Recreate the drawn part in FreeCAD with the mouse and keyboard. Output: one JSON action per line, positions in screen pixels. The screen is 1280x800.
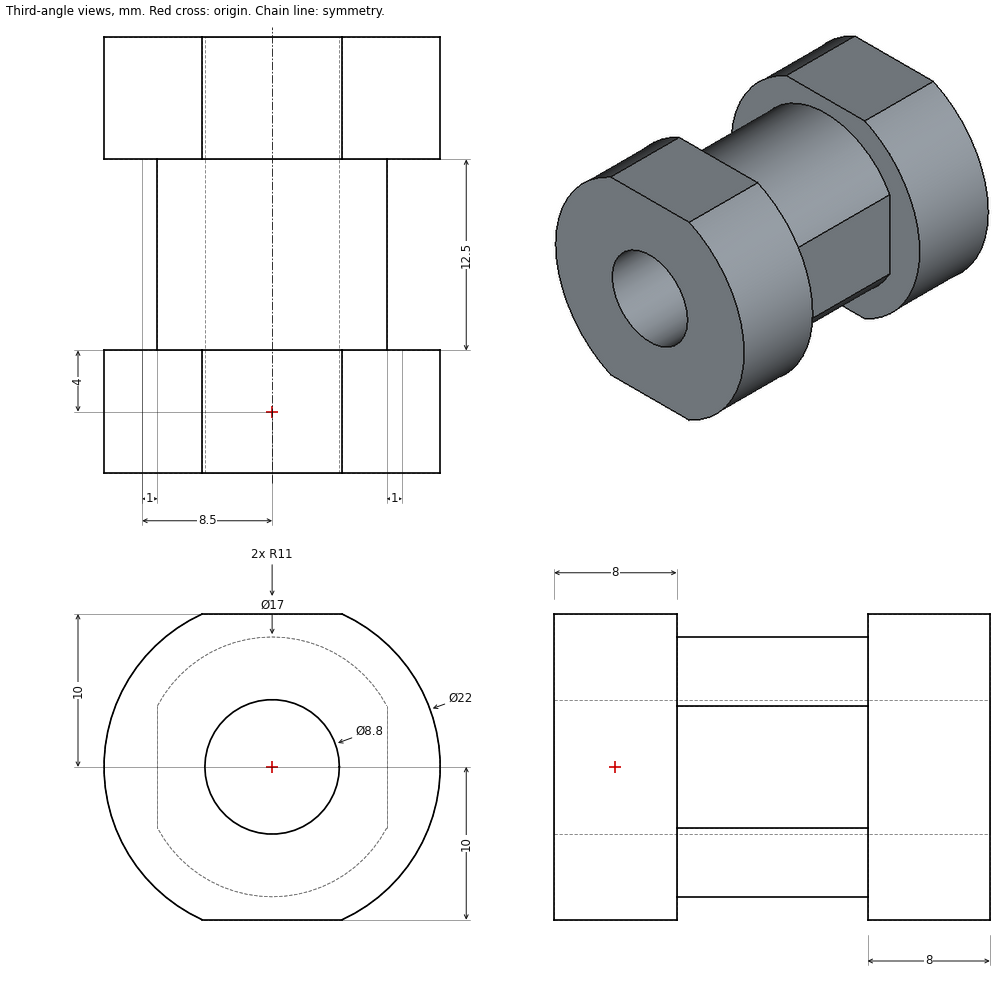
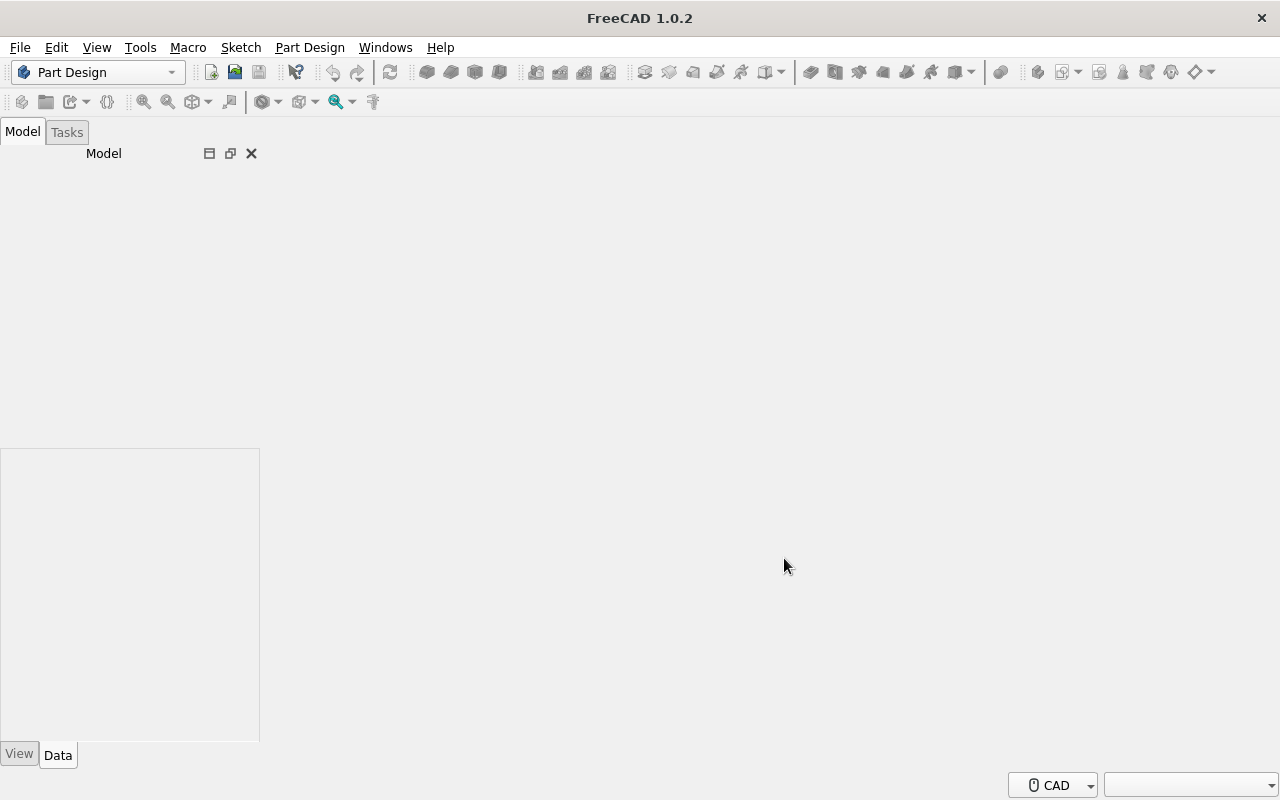
{"action": "left_click", "coordinate": [212, 72]}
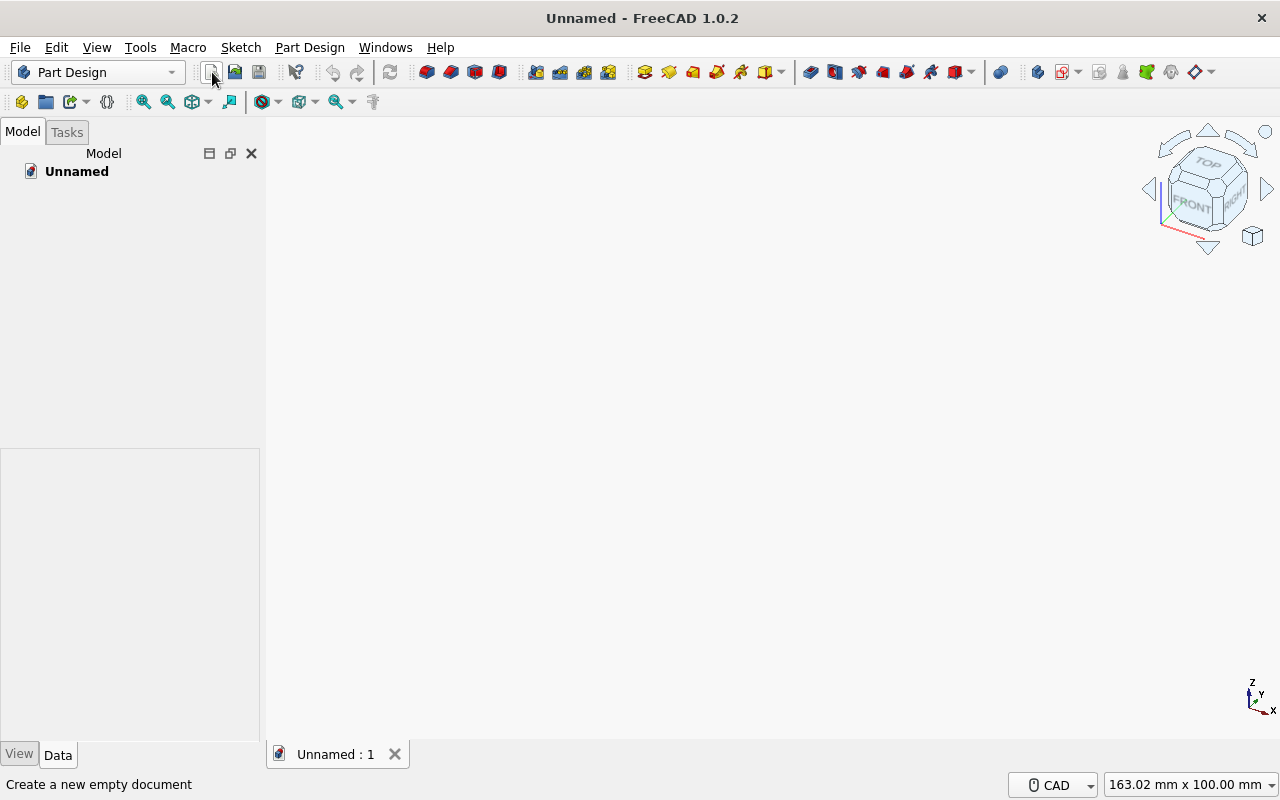
{"action": "left_click", "coordinate": [1062, 72]}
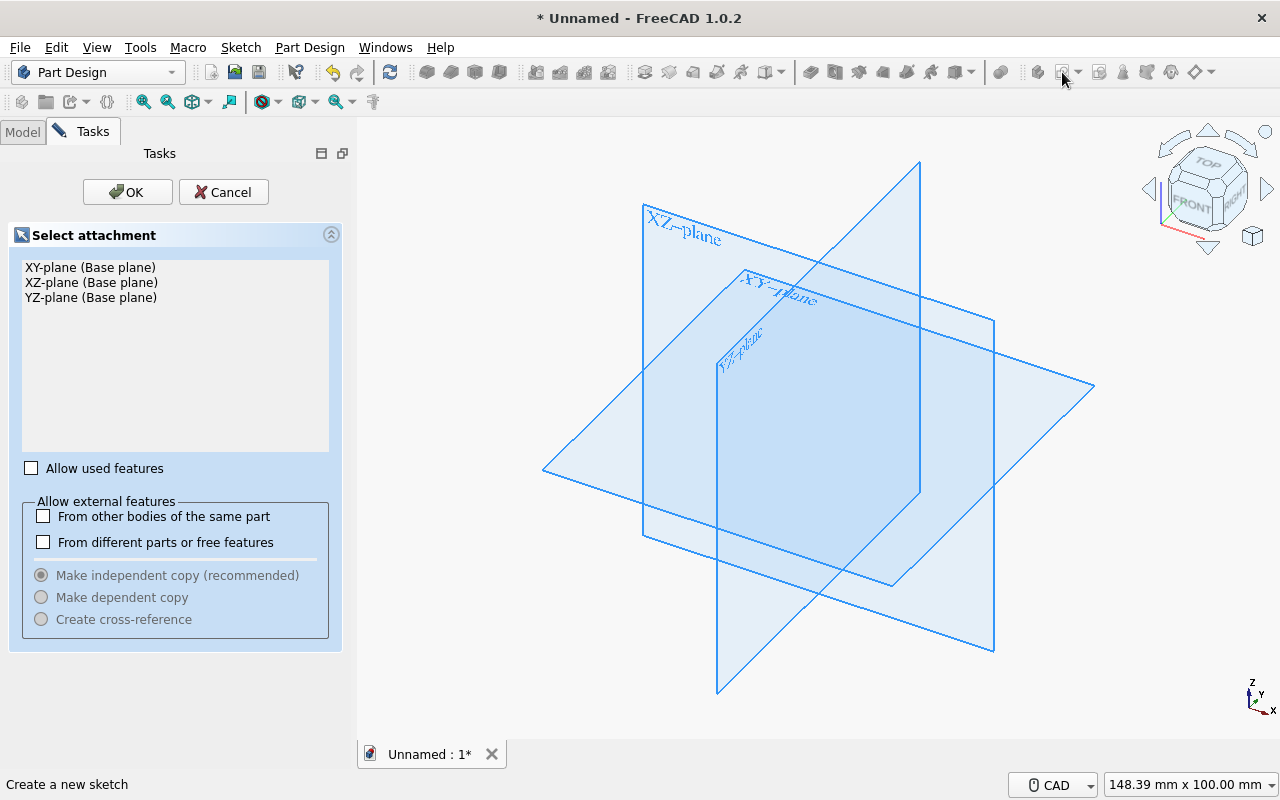
{"action": "left_click", "coordinate": [82, 282]}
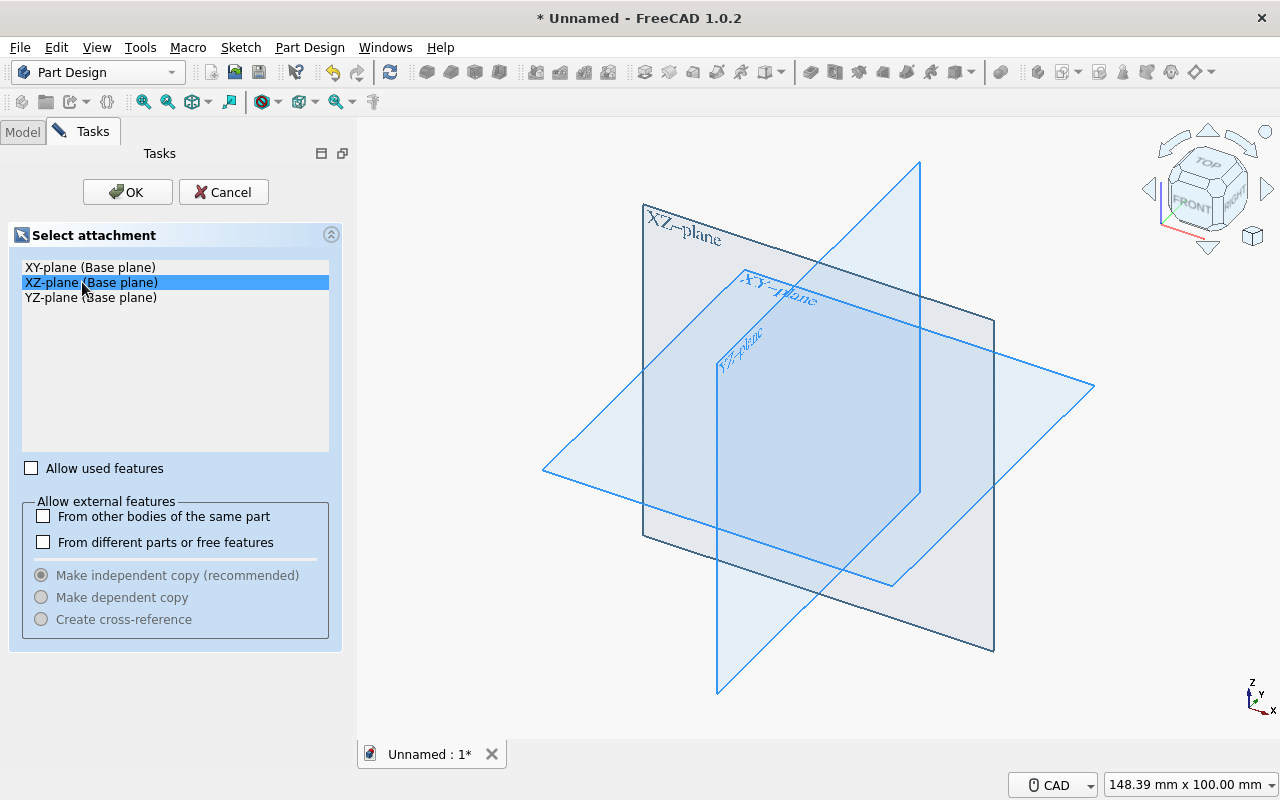
{"action": "left_click", "coordinate": [128, 192]}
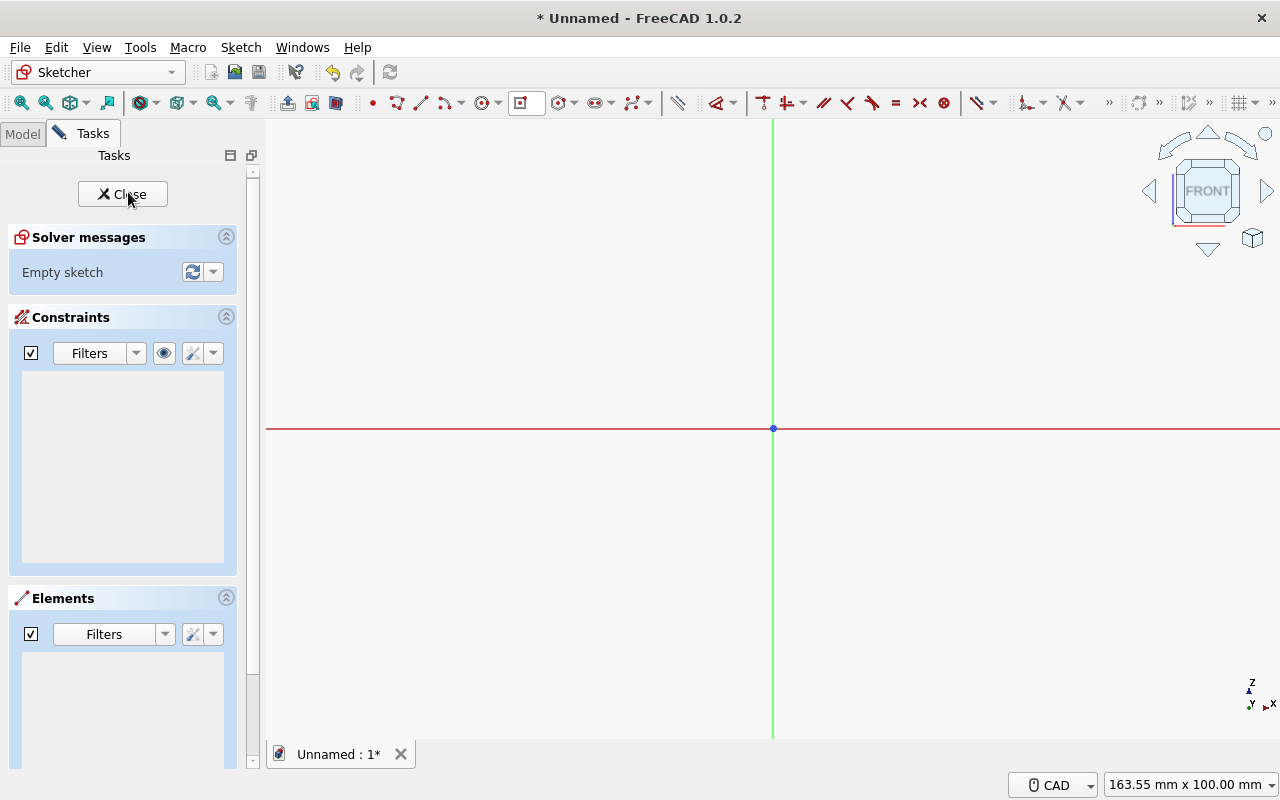
{"action": "scroll", "coordinate": [813, 429], "scroll_direction": "up", "scroll_amount": 5}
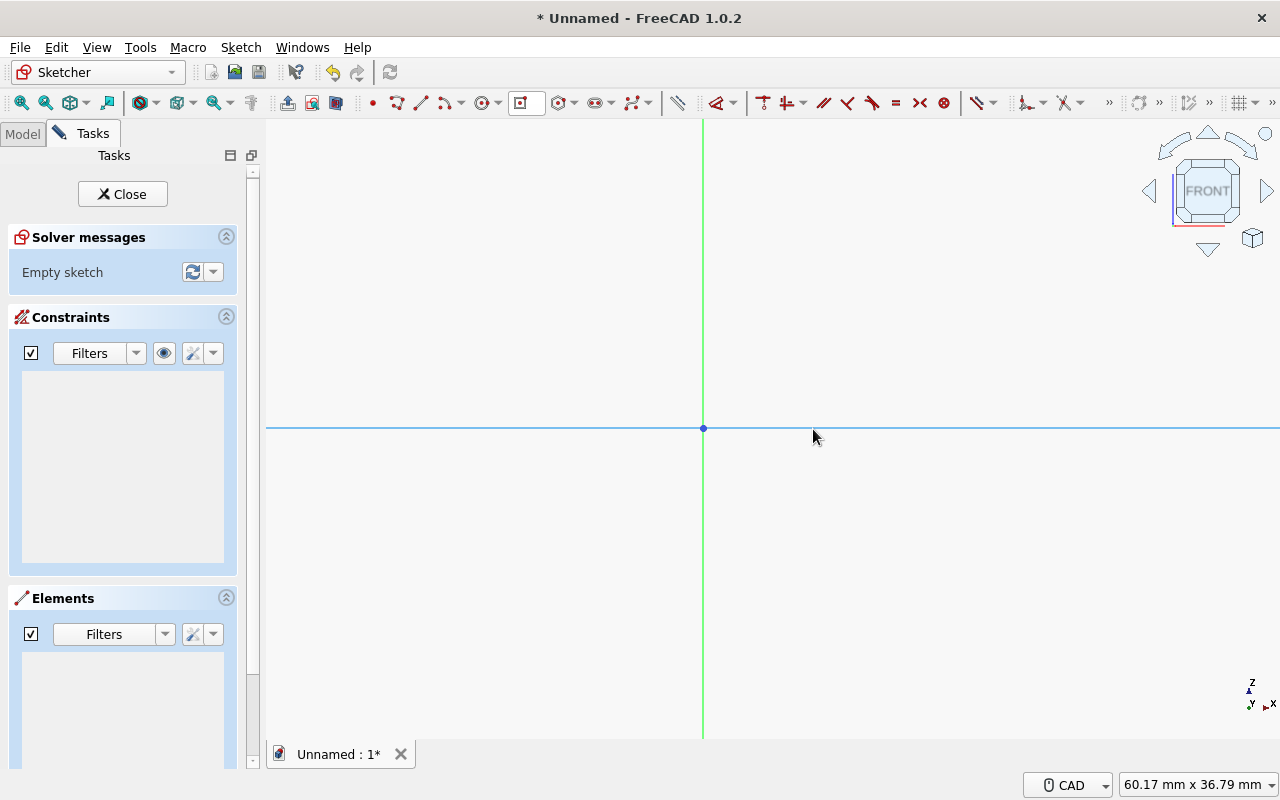
{"action": "left_click", "coordinate": [482, 104]}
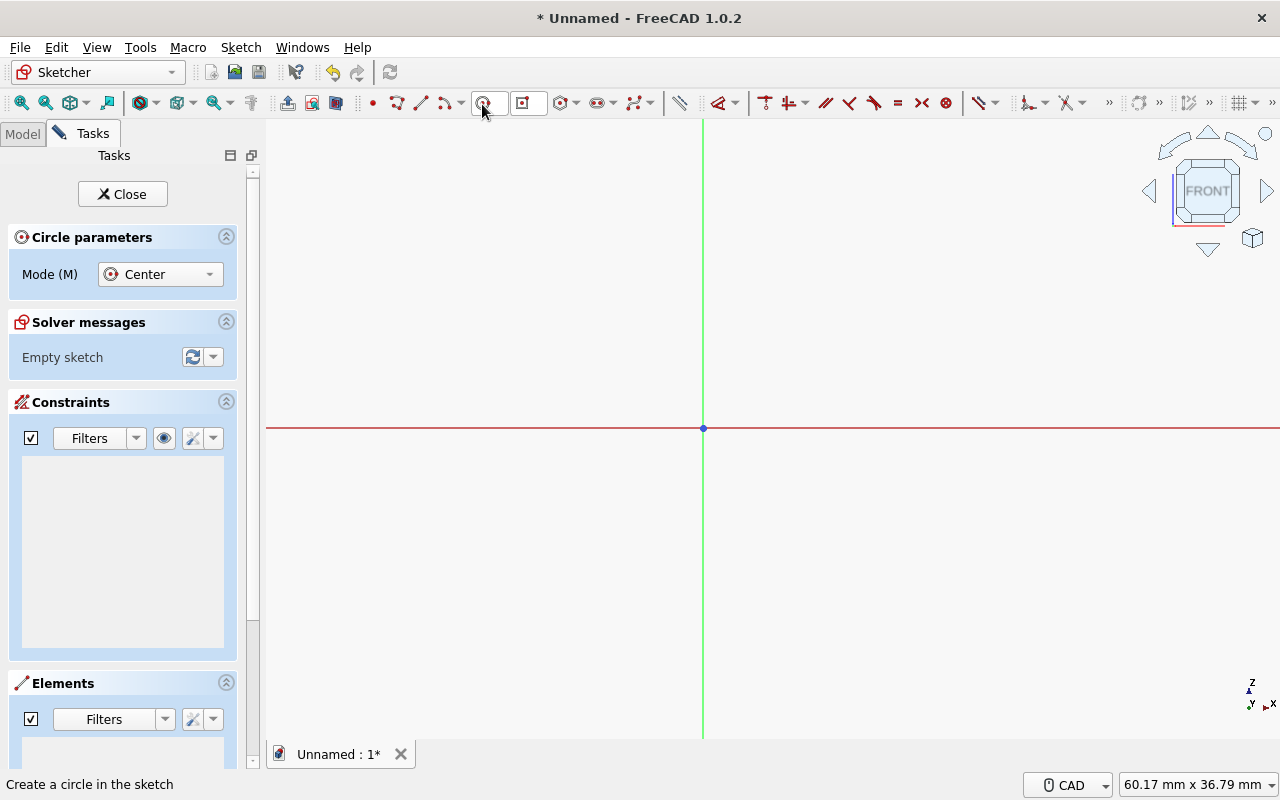
{"action": "left_click", "coordinate": [703, 428]}
{"action": "mouse_move", "coordinate": [834, 297]}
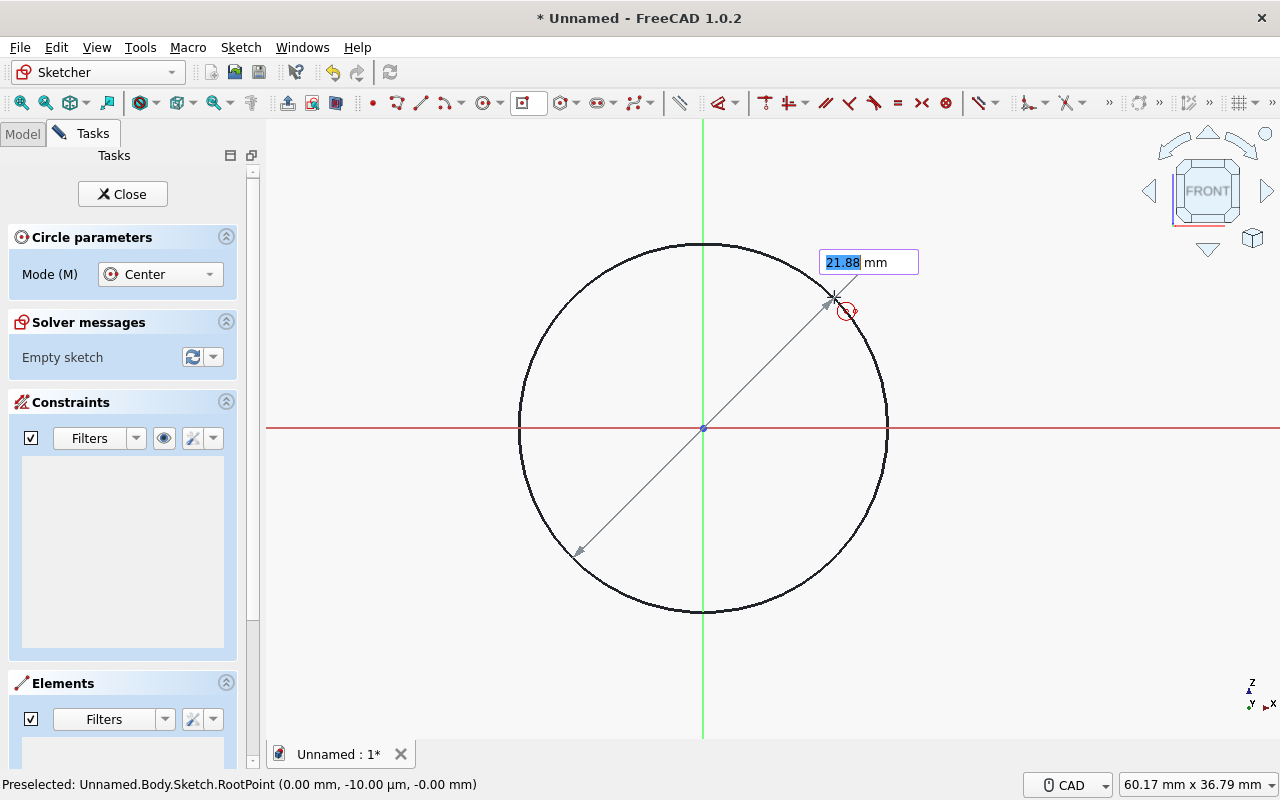
{"action": "type", "text": "22"}
{"action": "key", "text": "Return"}
{"action": "key", "text": "Escape"}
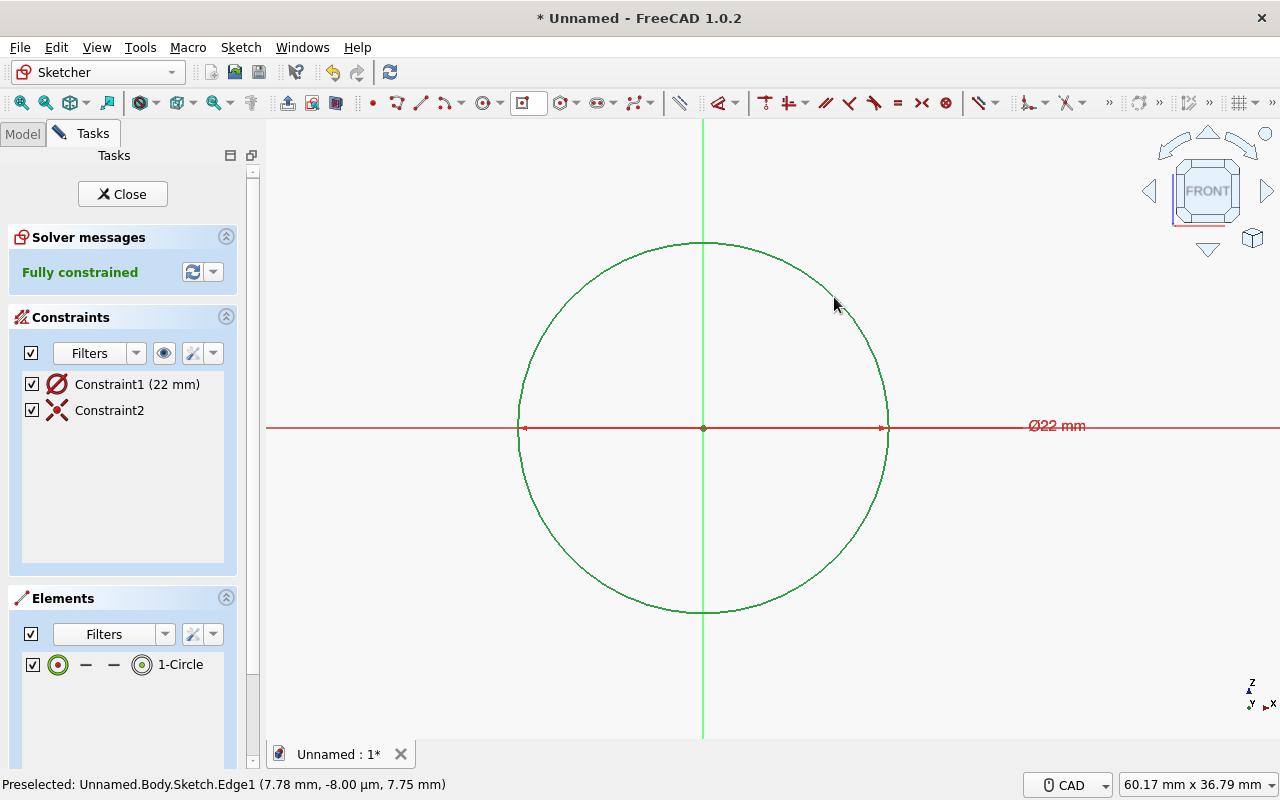
{"action": "left_click", "coordinate": [123, 194]}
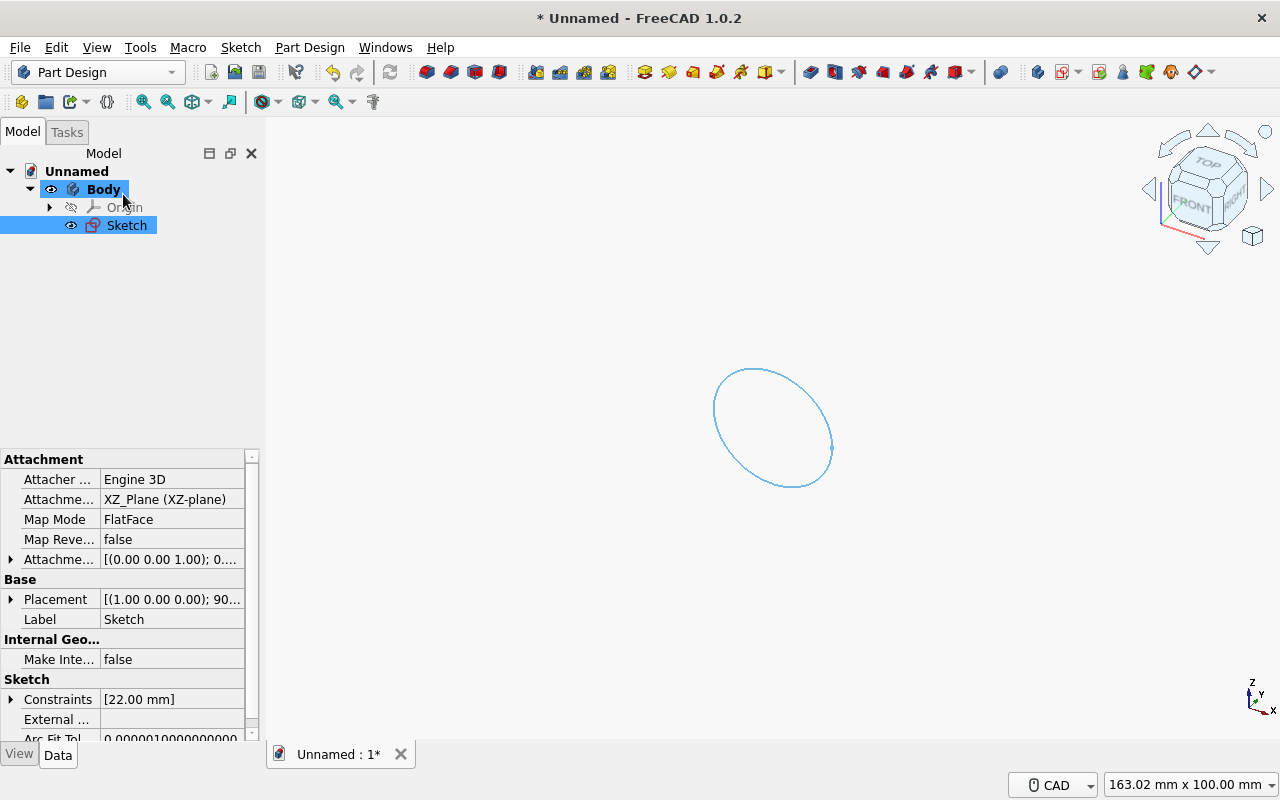
{"action": "left_click", "coordinate": [646, 72]}